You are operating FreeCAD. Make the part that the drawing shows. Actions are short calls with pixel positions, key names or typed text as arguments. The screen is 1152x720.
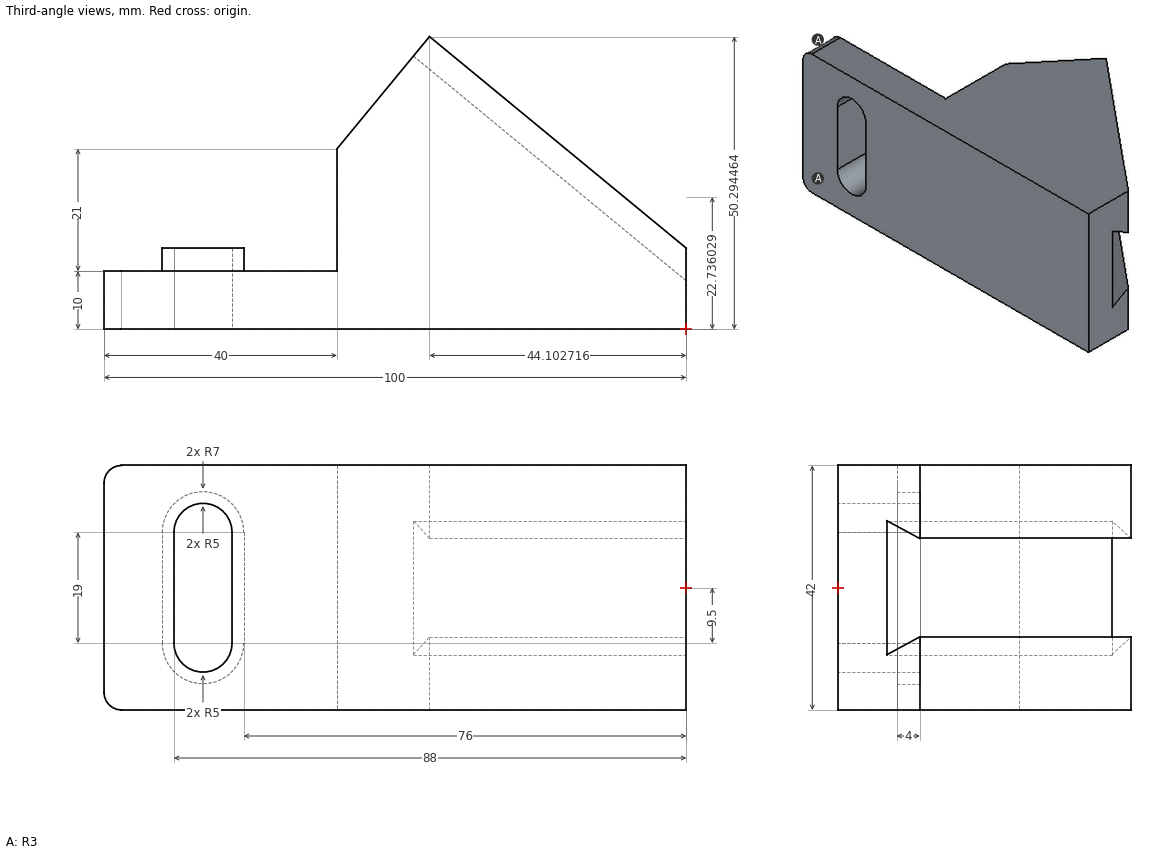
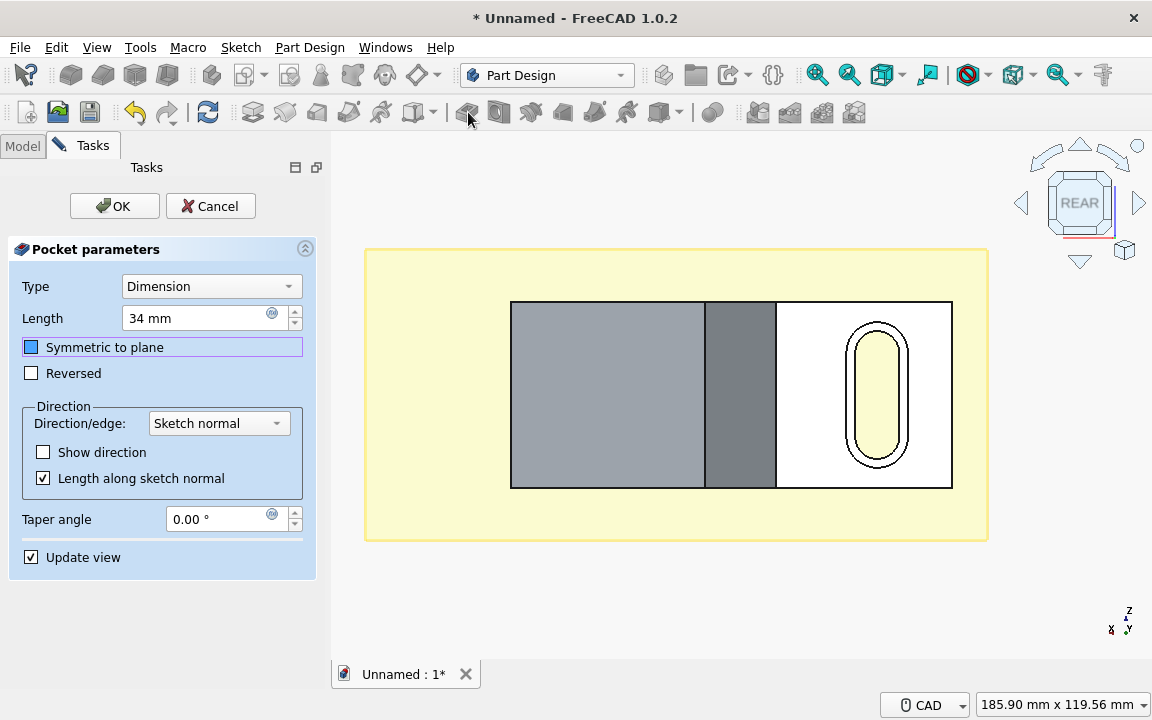
click(115, 206)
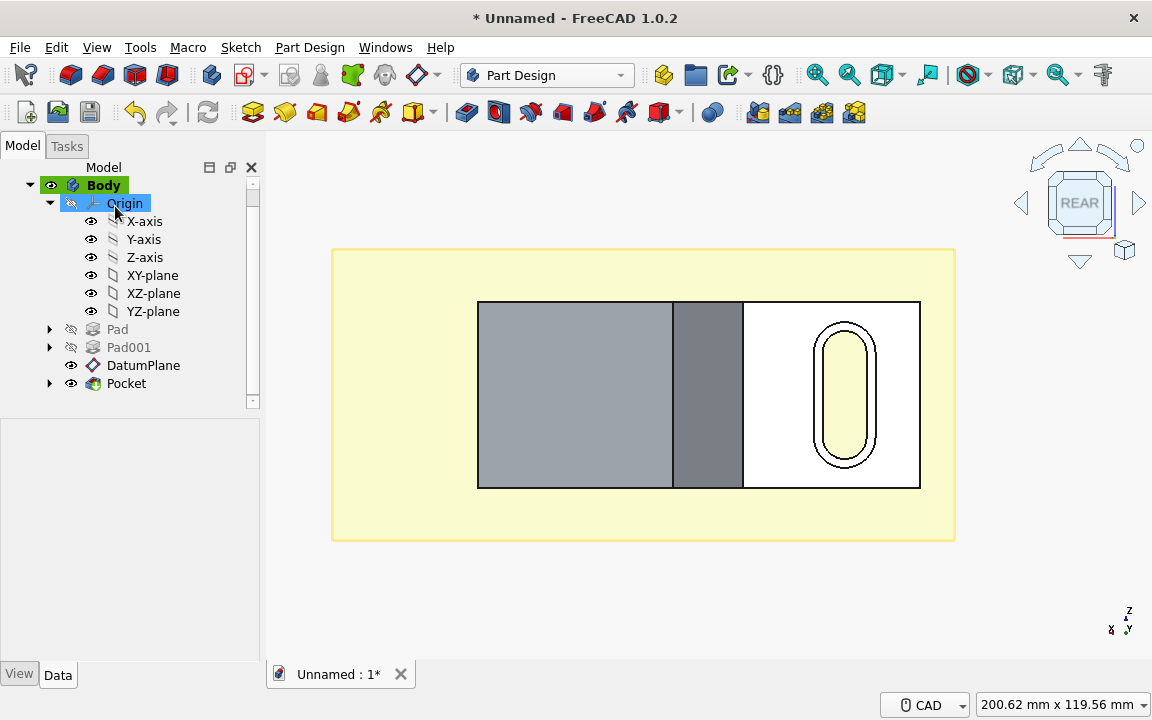
click(116, 365)
key(space)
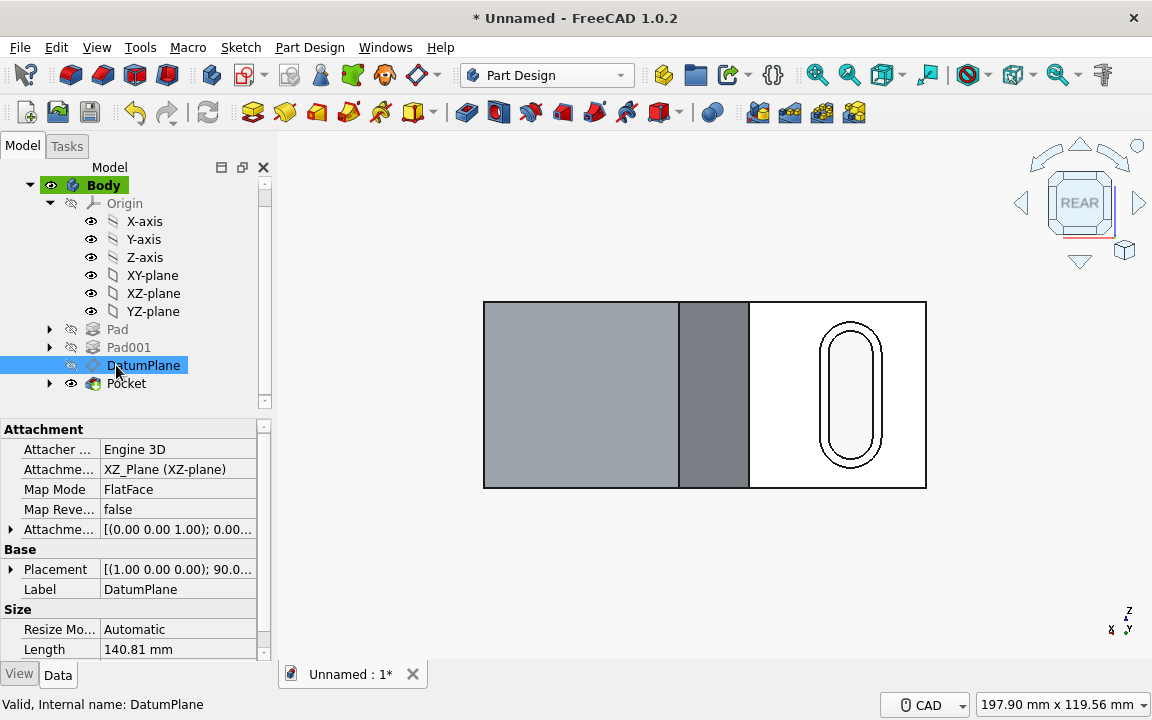
click(714, 368)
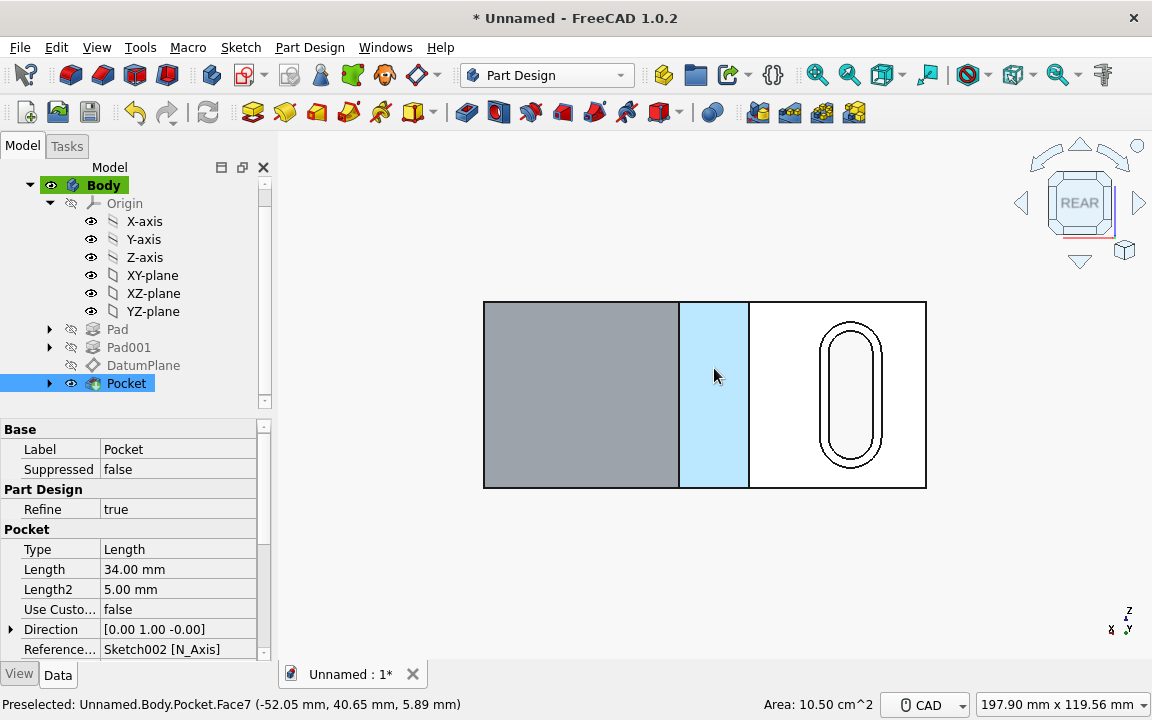
click(244, 76)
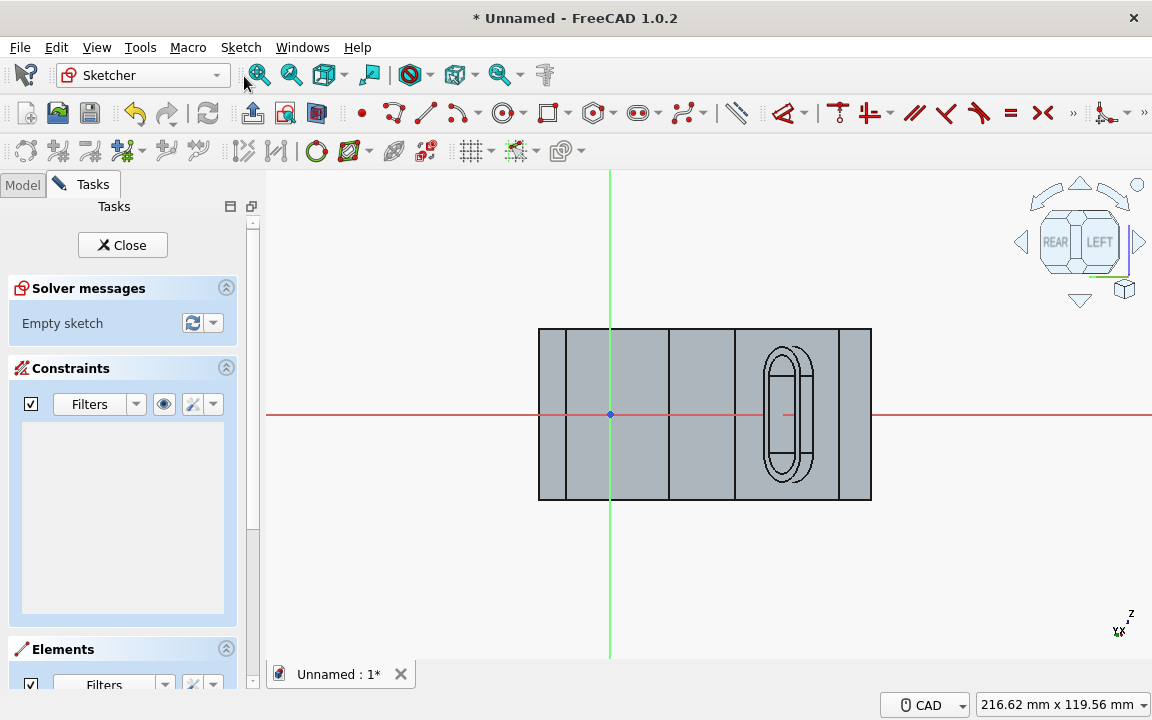
scroll(494, 415, up, 3)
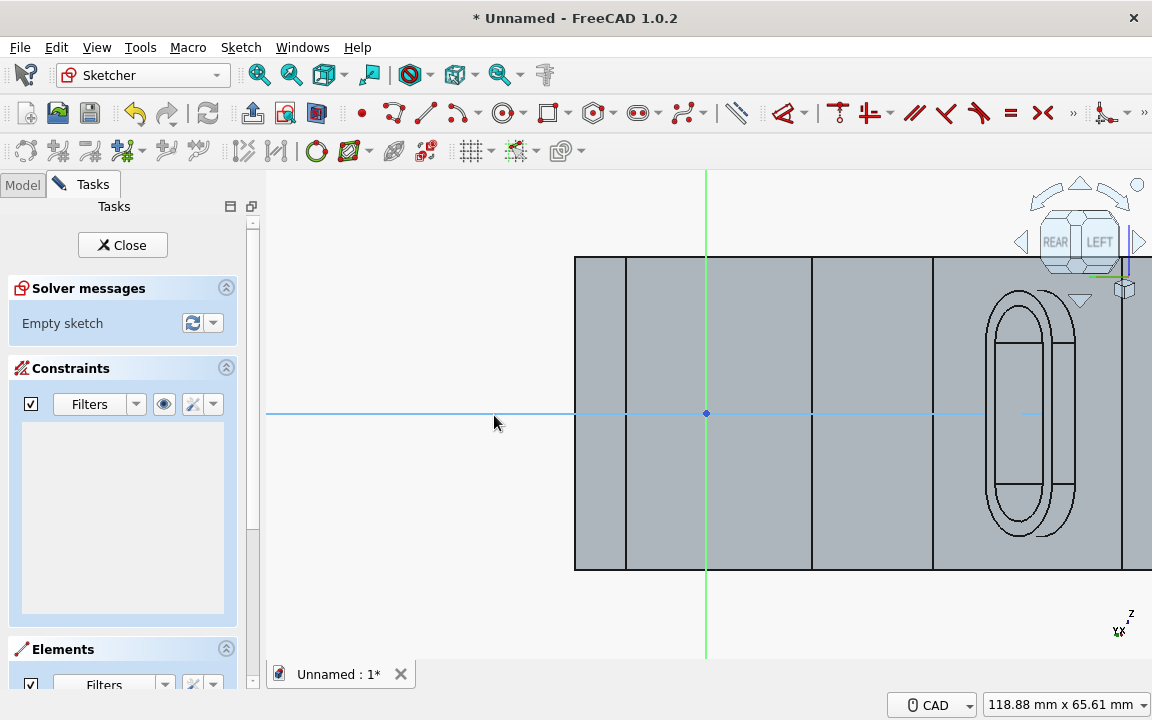
key(g)
key(m)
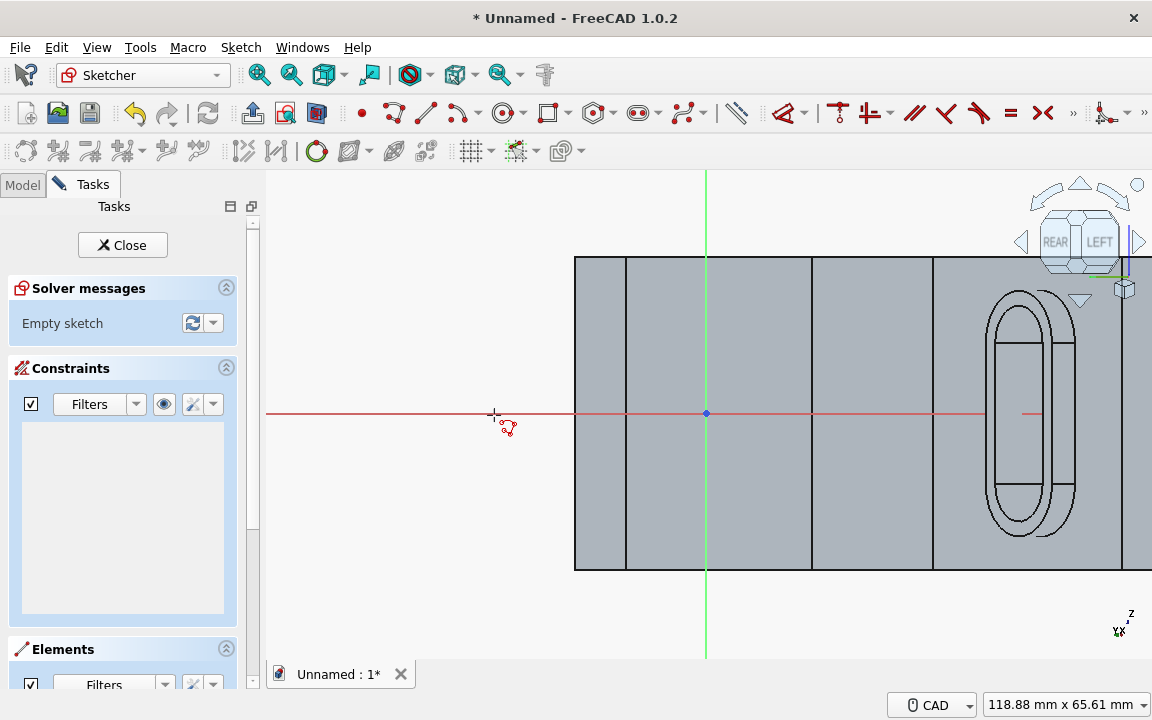
click(658, 499)
click(658, 328)
click(626, 351)
click(626, 257)
click(575, 257)
click(575, 570)
click(626, 570)
click(626, 477)
click(658, 500)
key(Escape)
key(Escape)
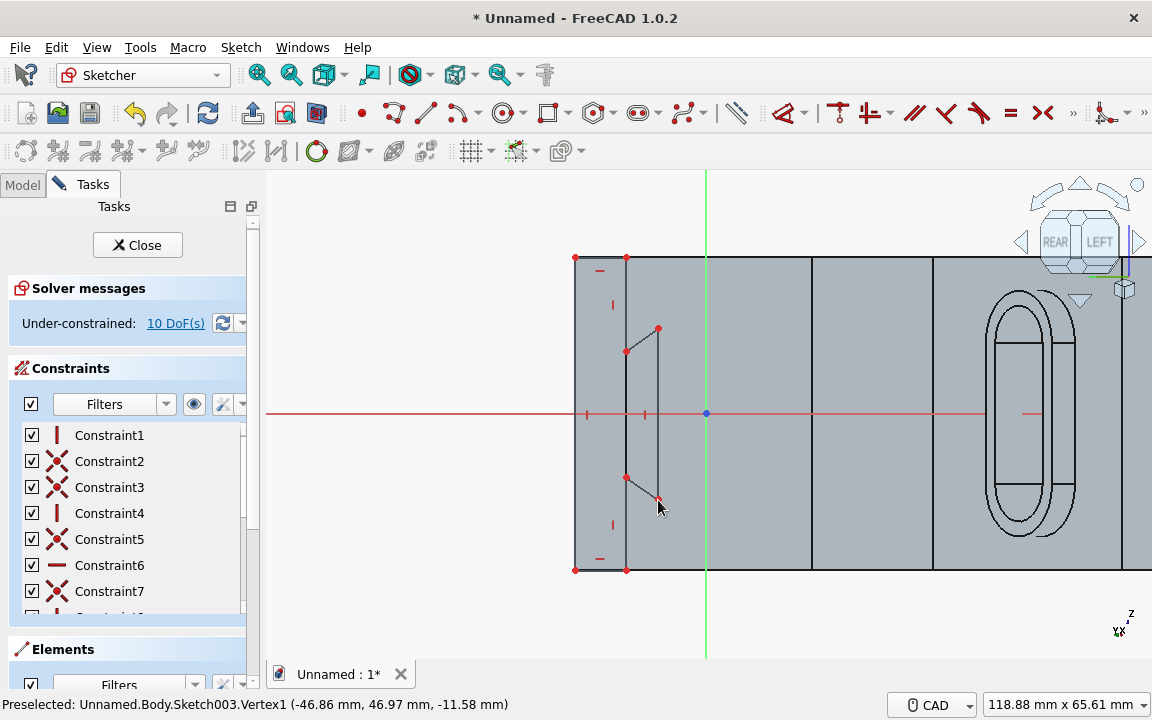
click(626, 258)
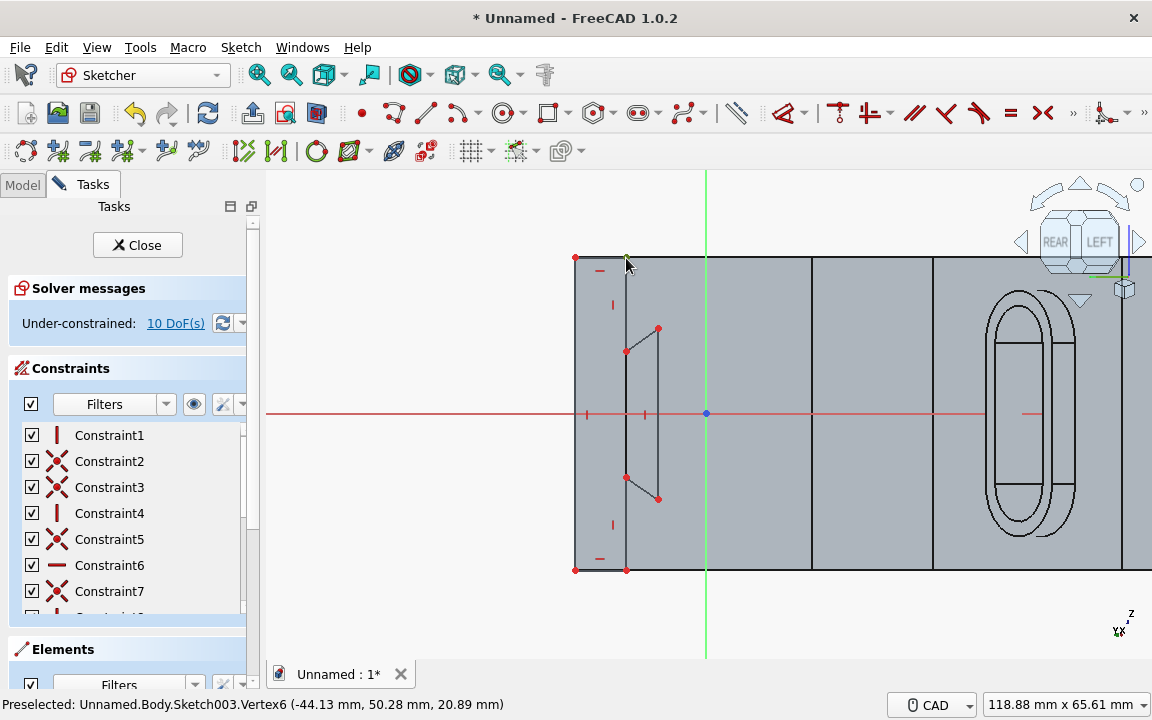
click(626, 571)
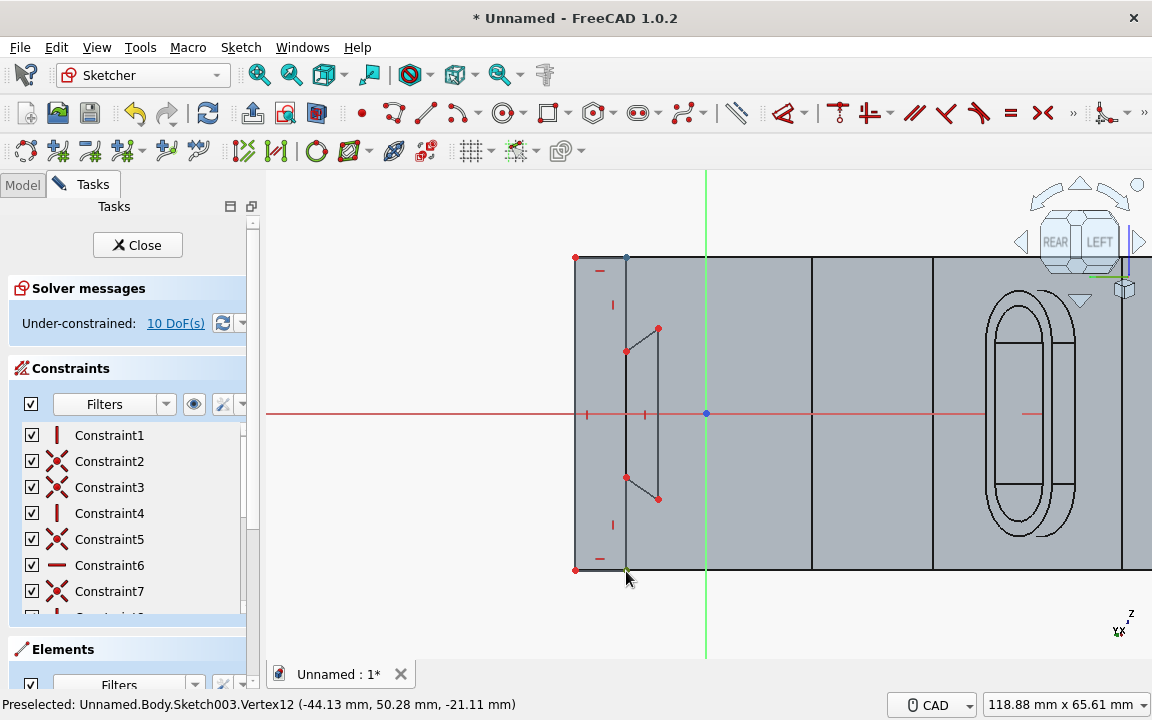
click(343, 414)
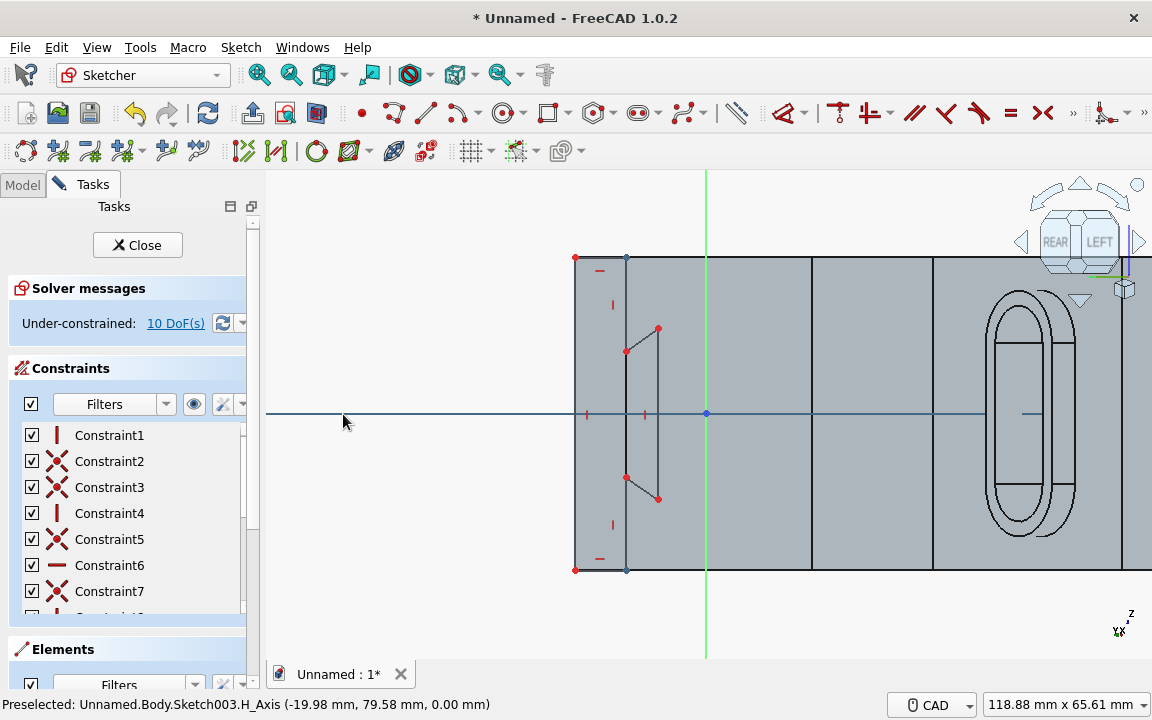
key(s)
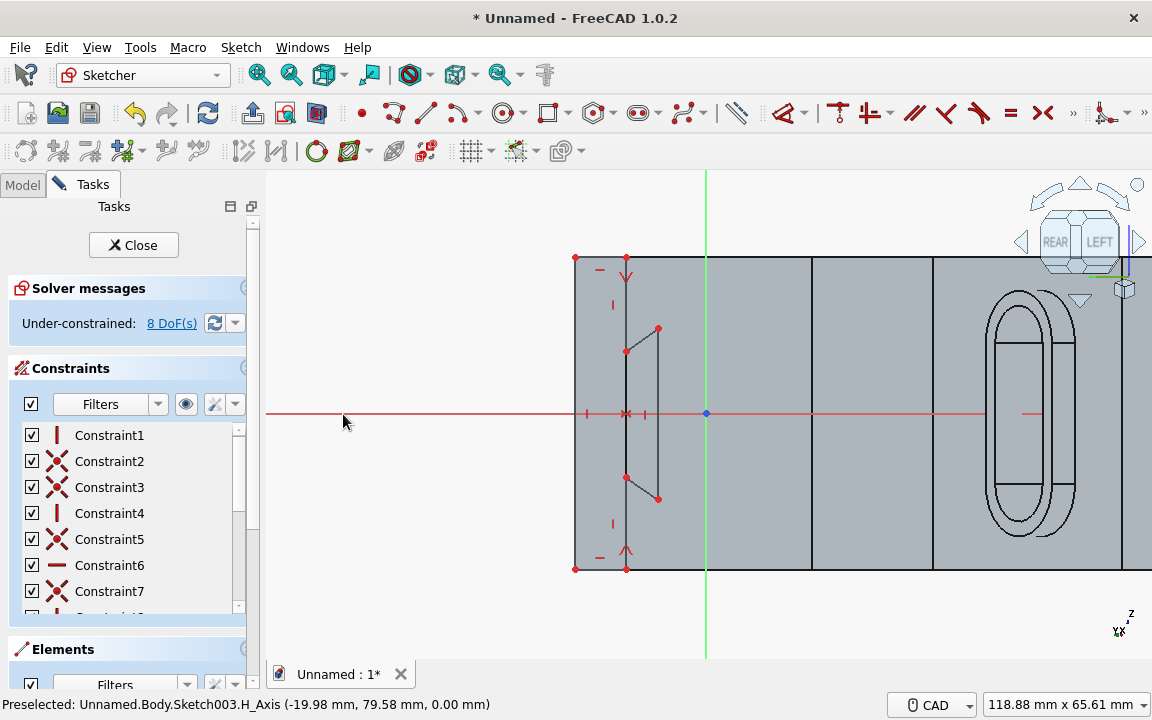
key(d)